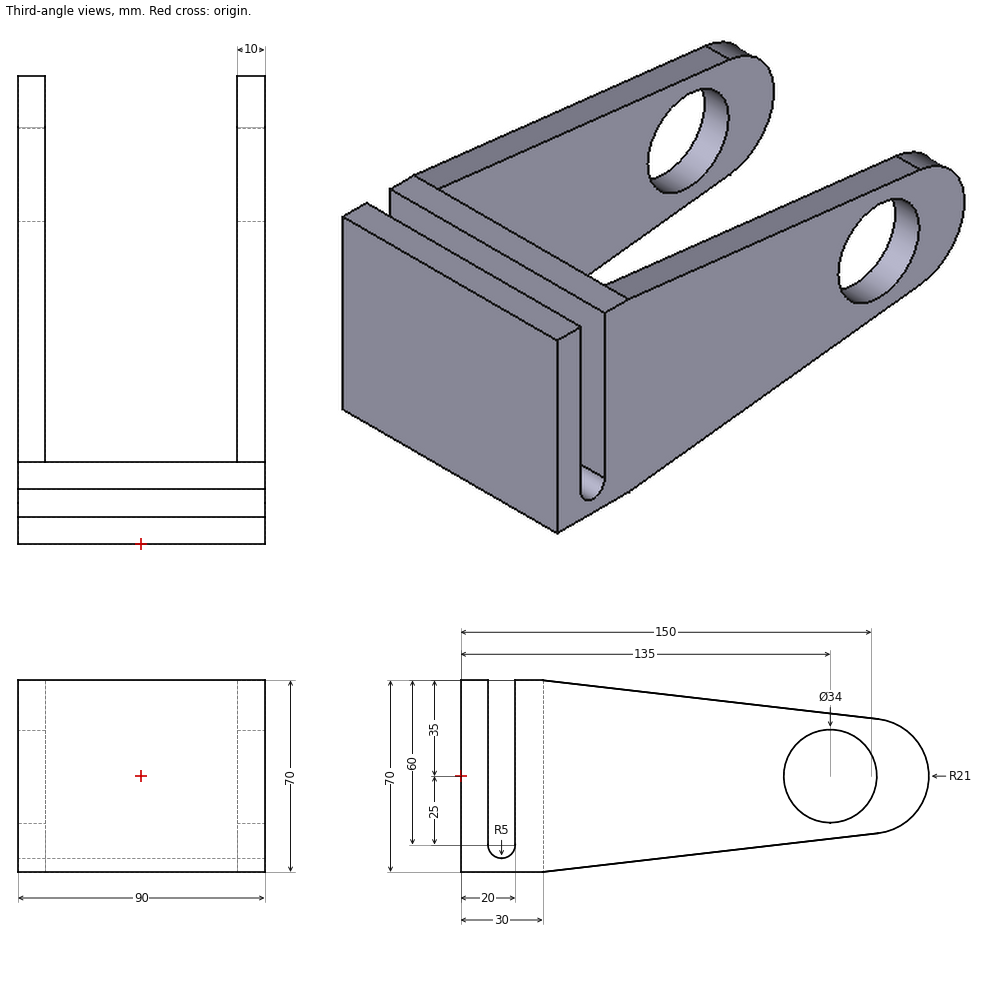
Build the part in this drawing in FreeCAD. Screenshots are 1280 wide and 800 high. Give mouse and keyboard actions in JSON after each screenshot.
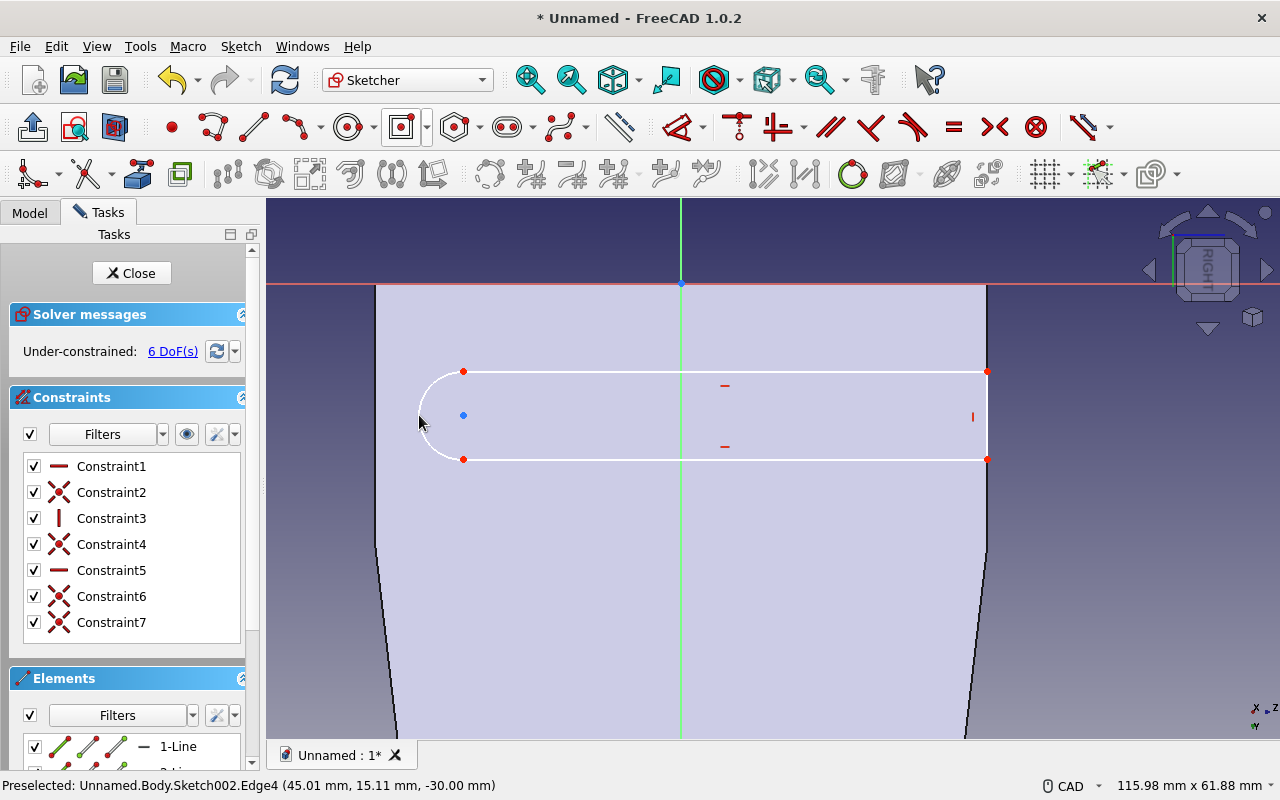
{"action": "left_click", "coordinate": [620, 460]}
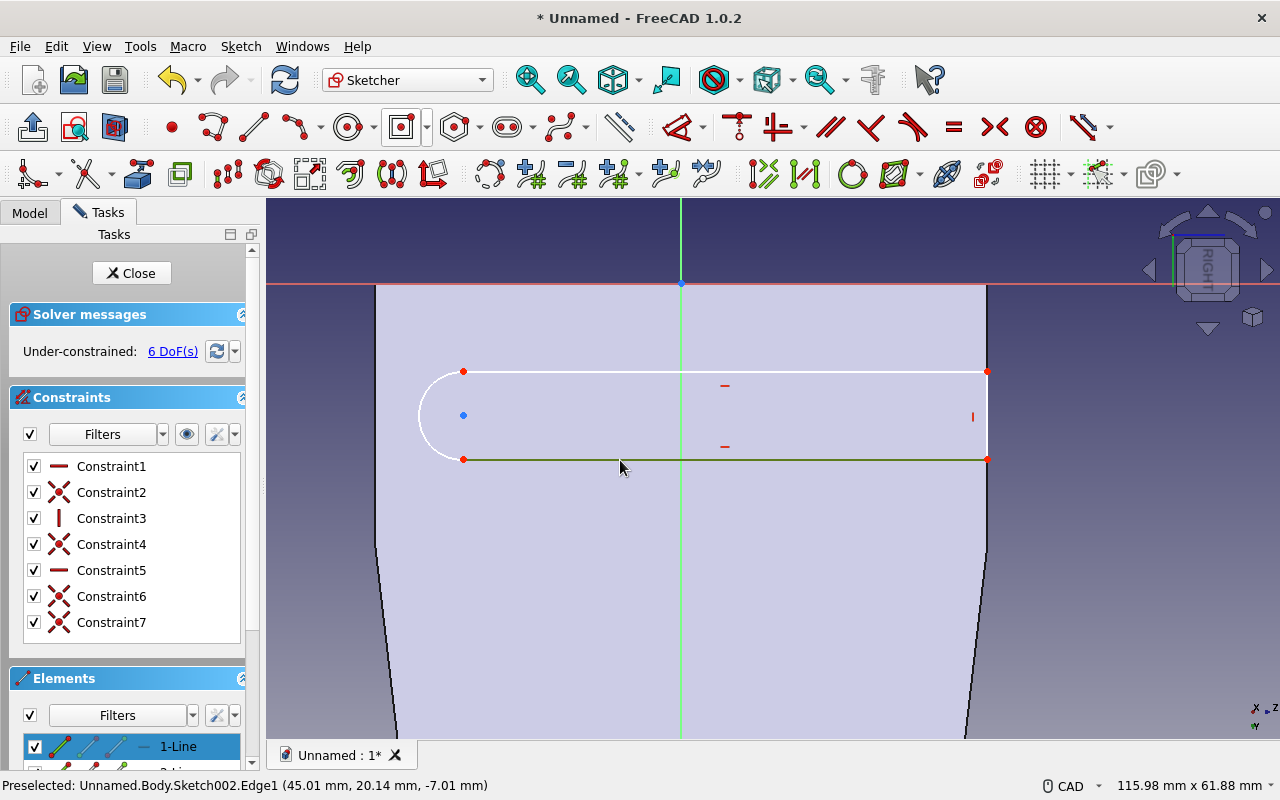
{"action": "left_click", "coordinate": [427, 390]}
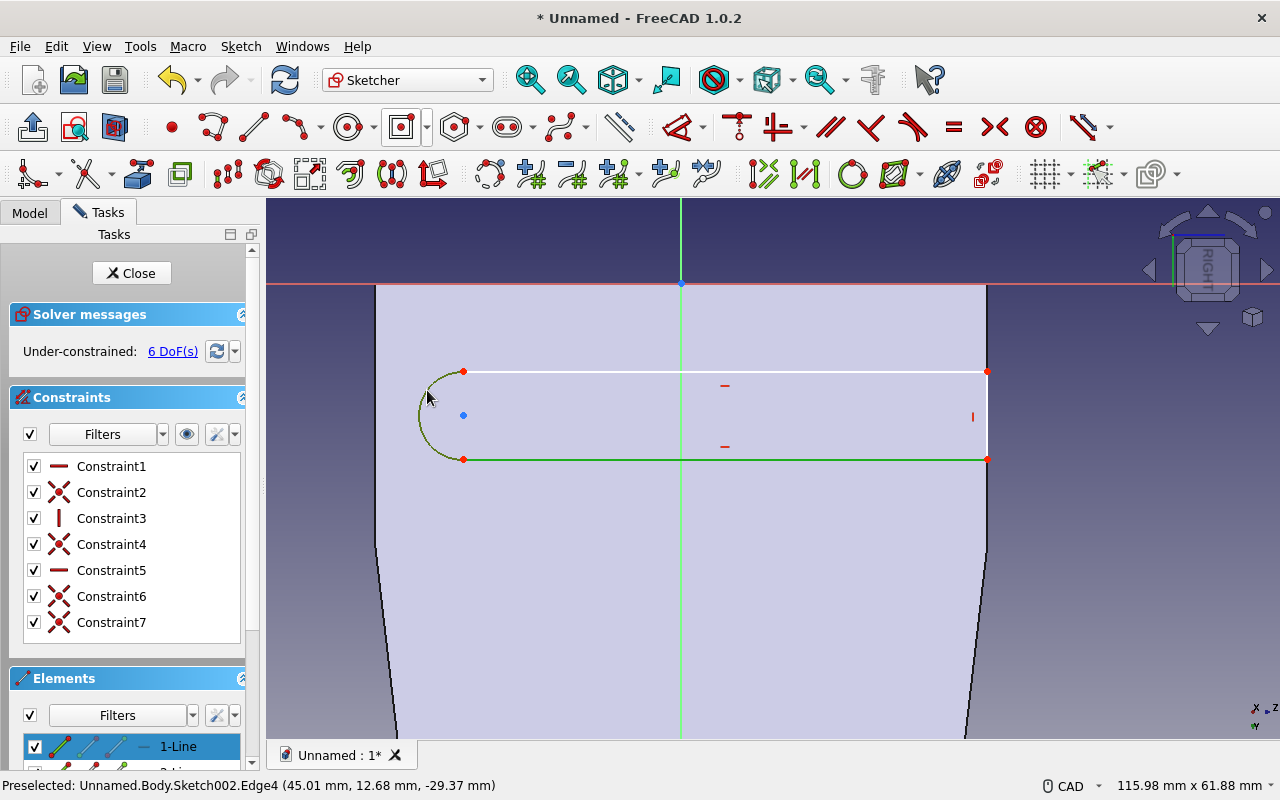
{"action": "left_click", "coordinate": [913, 128]}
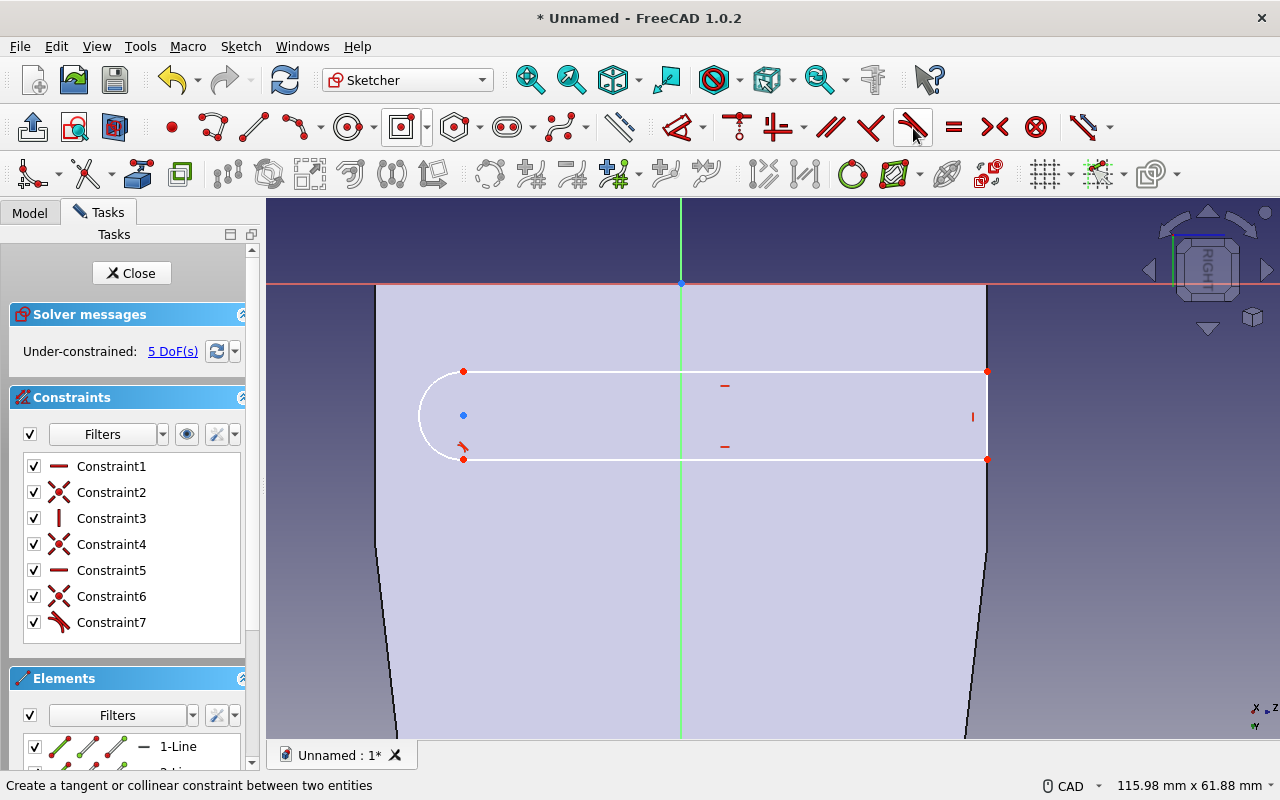
{"action": "left_click", "coordinate": [830, 372]}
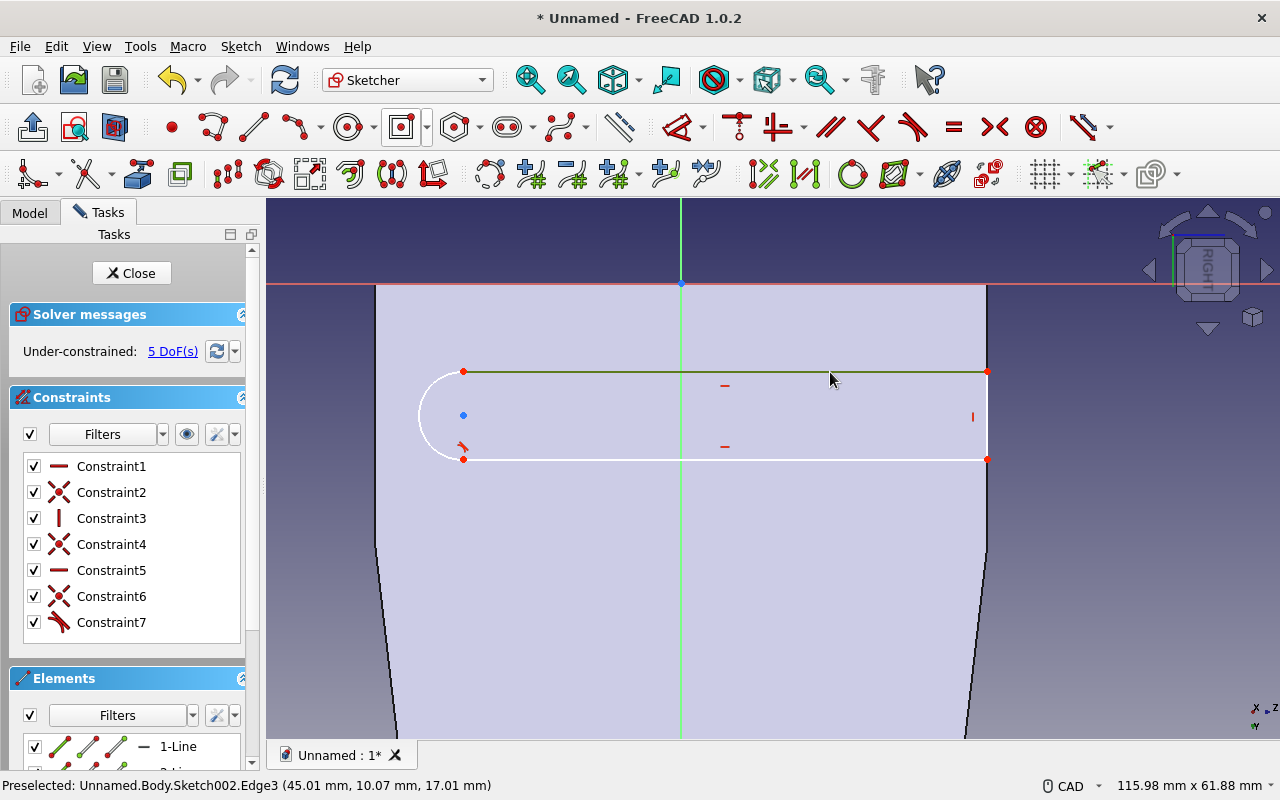
{"action": "left_click", "coordinate": [427, 390]}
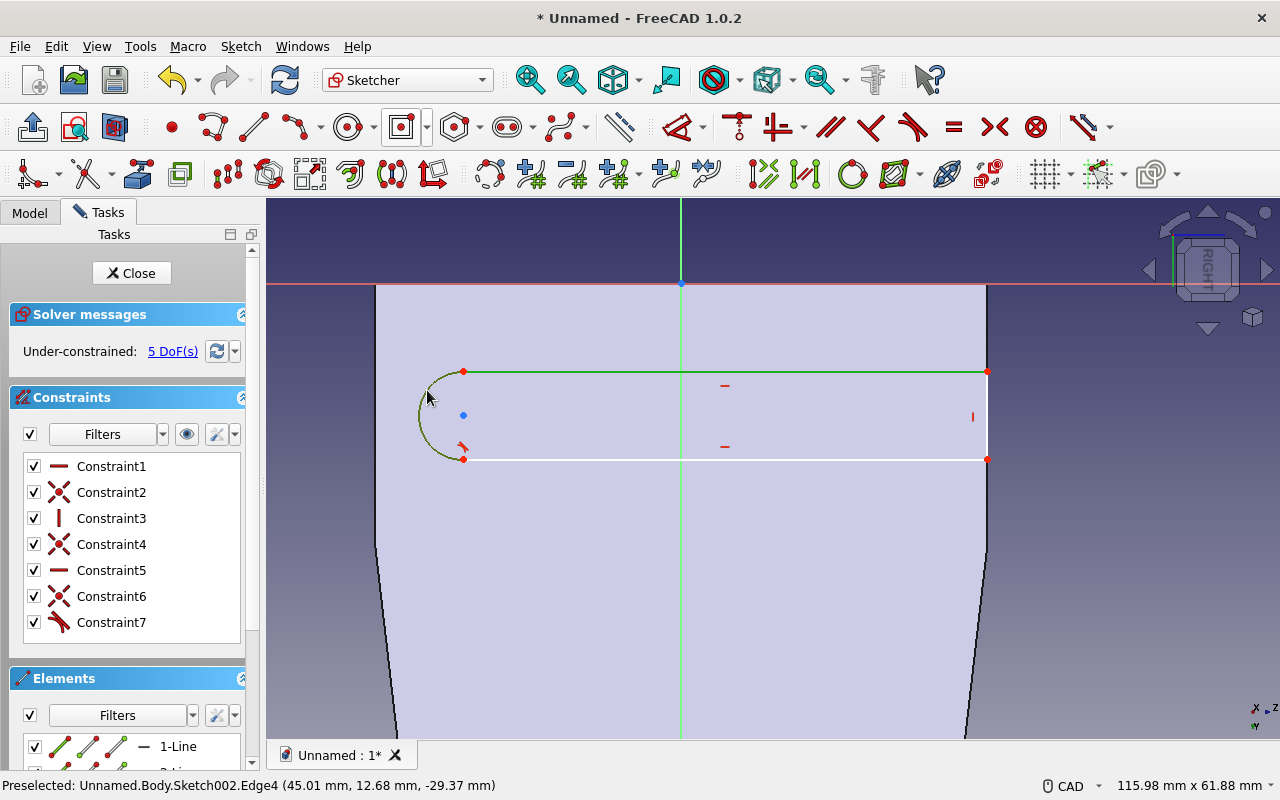
{"action": "left_click", "coordinate": [913, 128]}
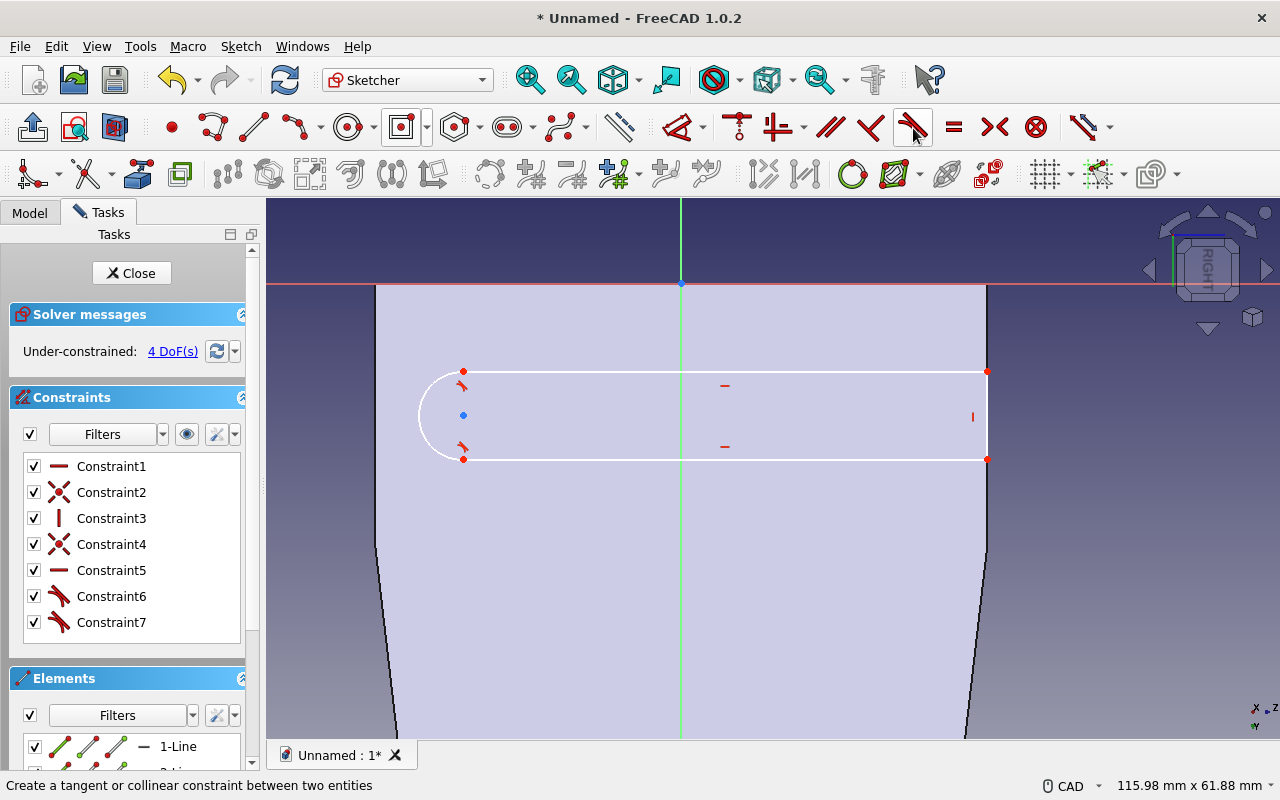
{"action": "left_click", "coordinate": [676, 128]}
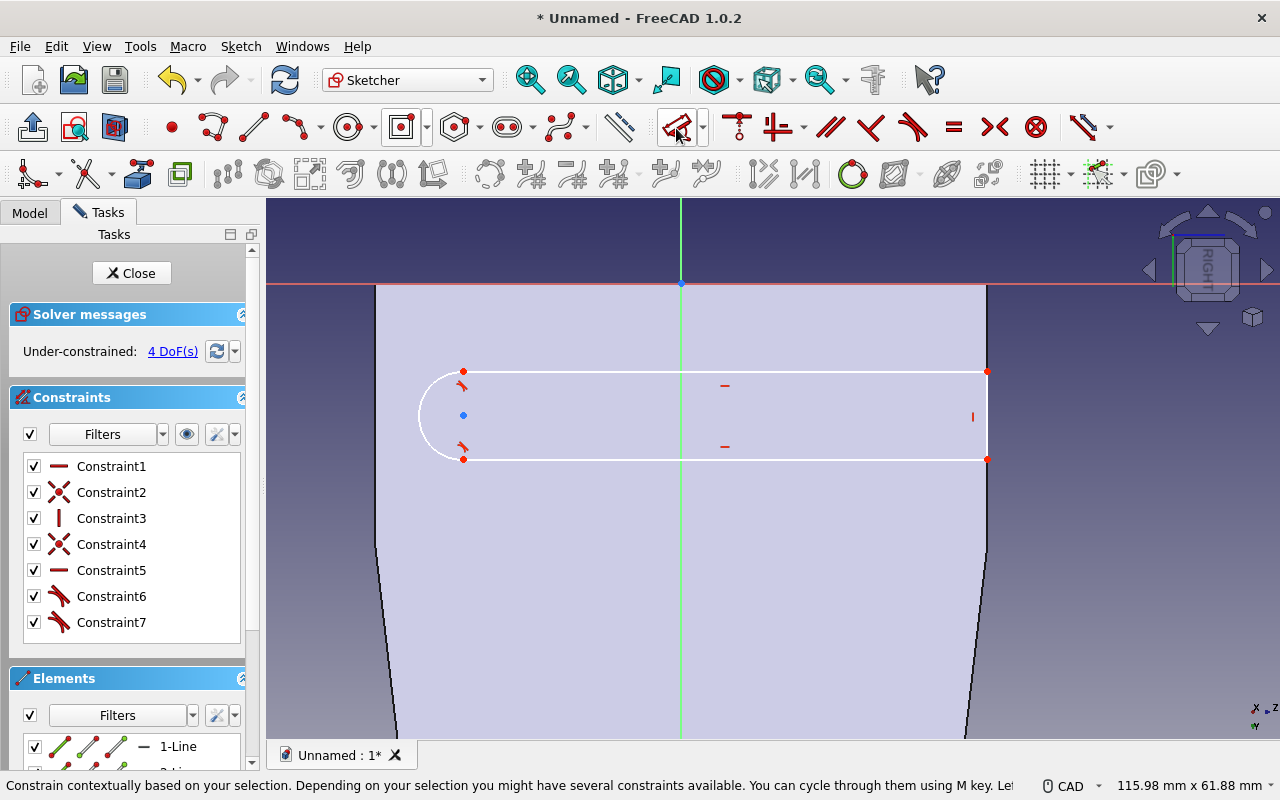
{"action": "left_click", "coordinate": [427, 390]}
{"action": "left_click", "coordinate": [401, 371]}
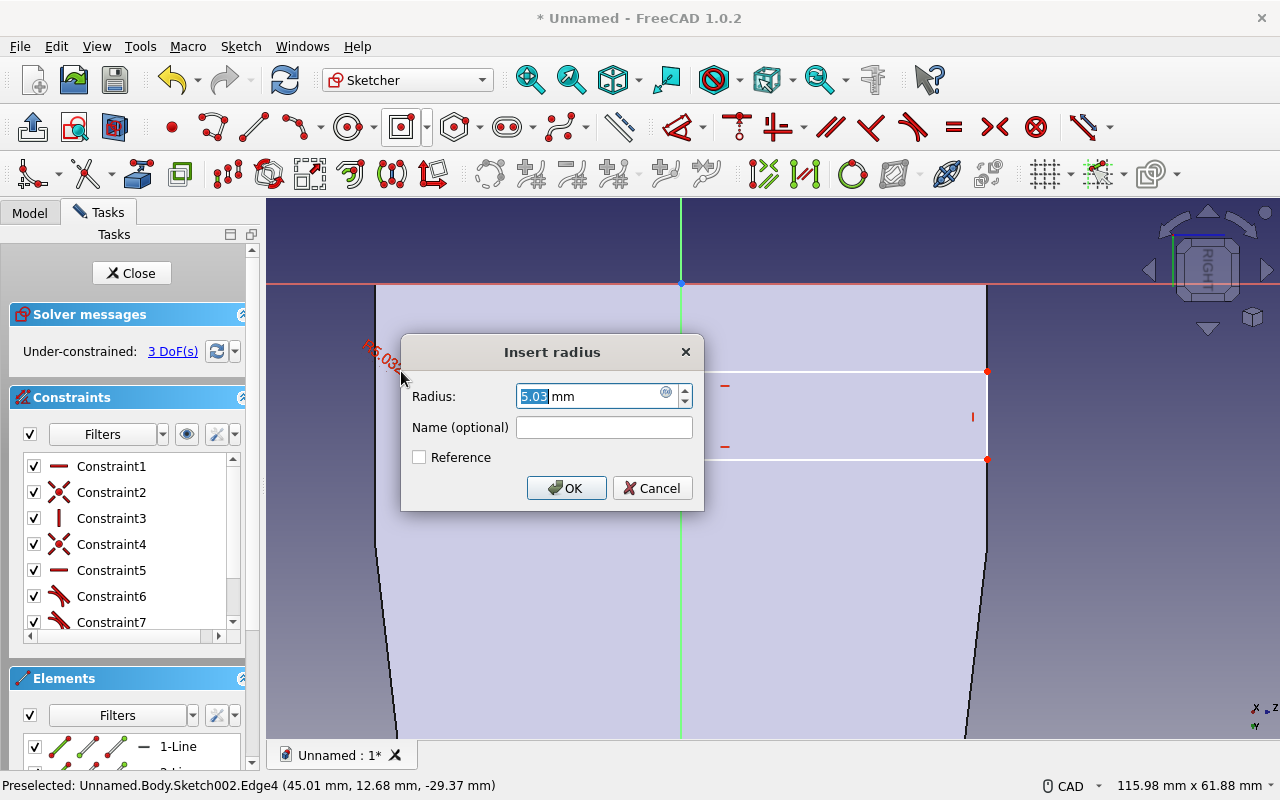
{"action": "type", "text": "5"}
{"action": "key", "text": "Return"}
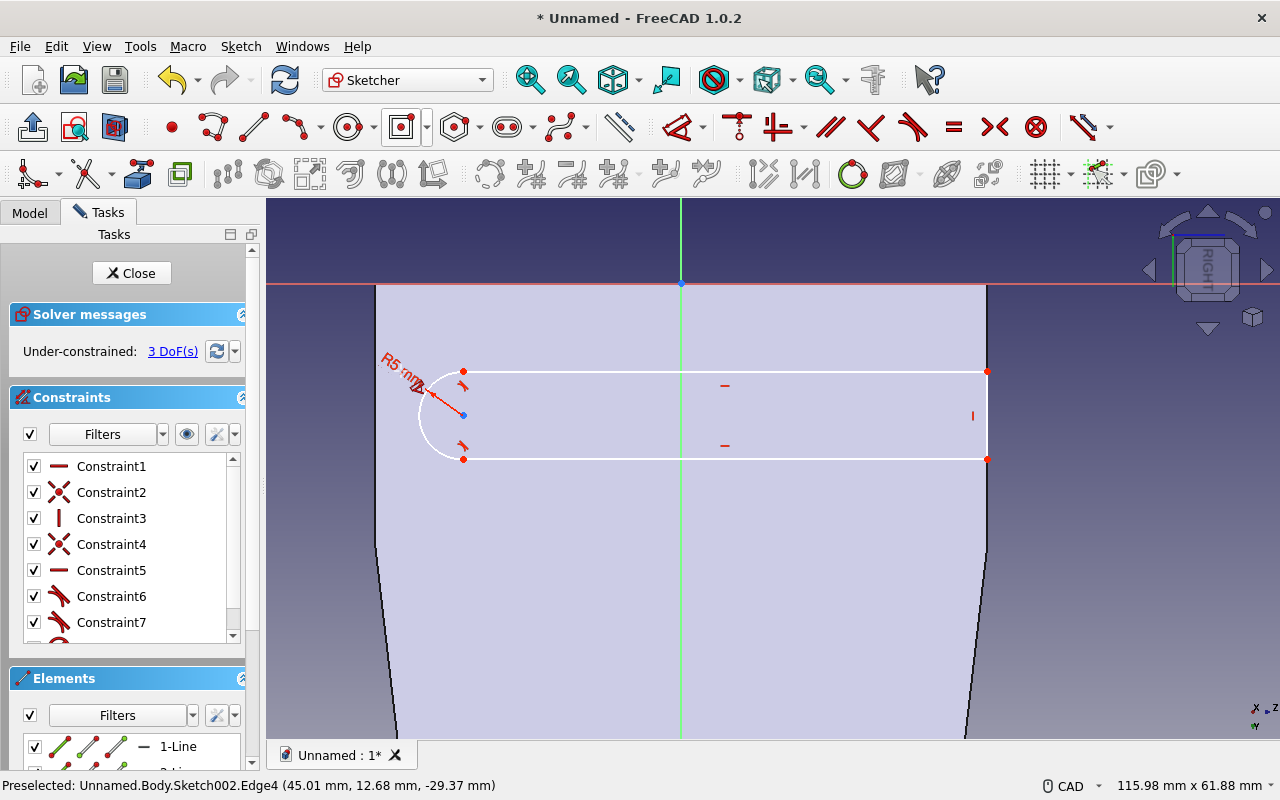
{"action": "left_click", "coordinate": [620, 459]}
{"action": "left_click", "coordinate": [725, 493]}